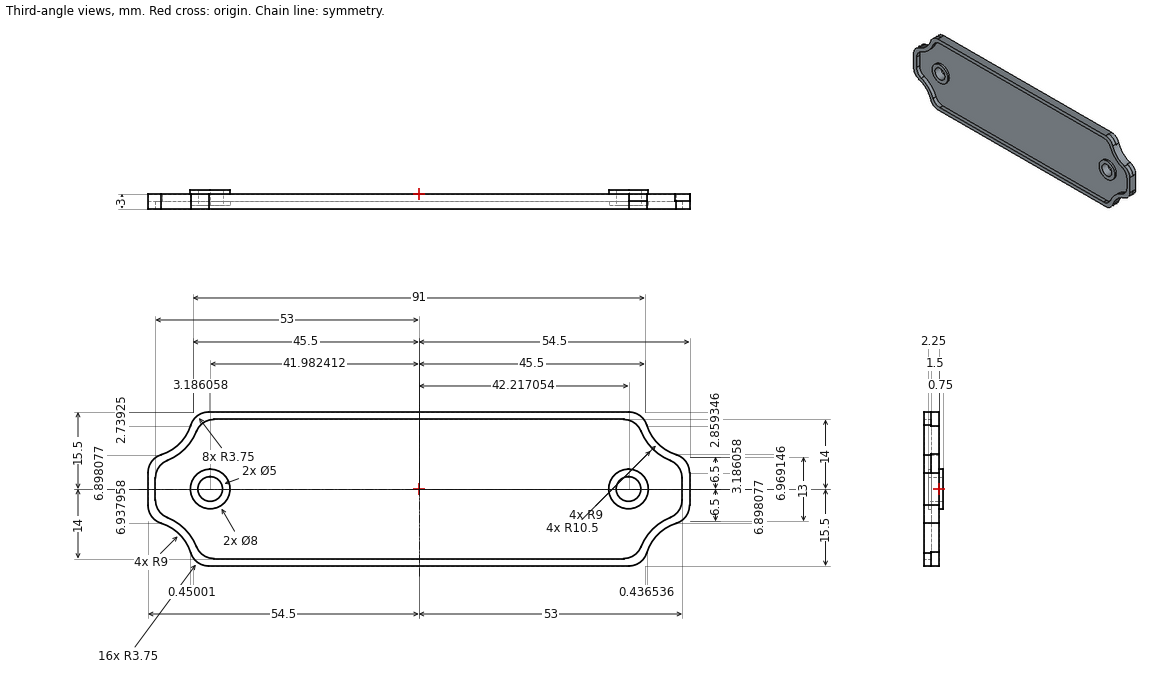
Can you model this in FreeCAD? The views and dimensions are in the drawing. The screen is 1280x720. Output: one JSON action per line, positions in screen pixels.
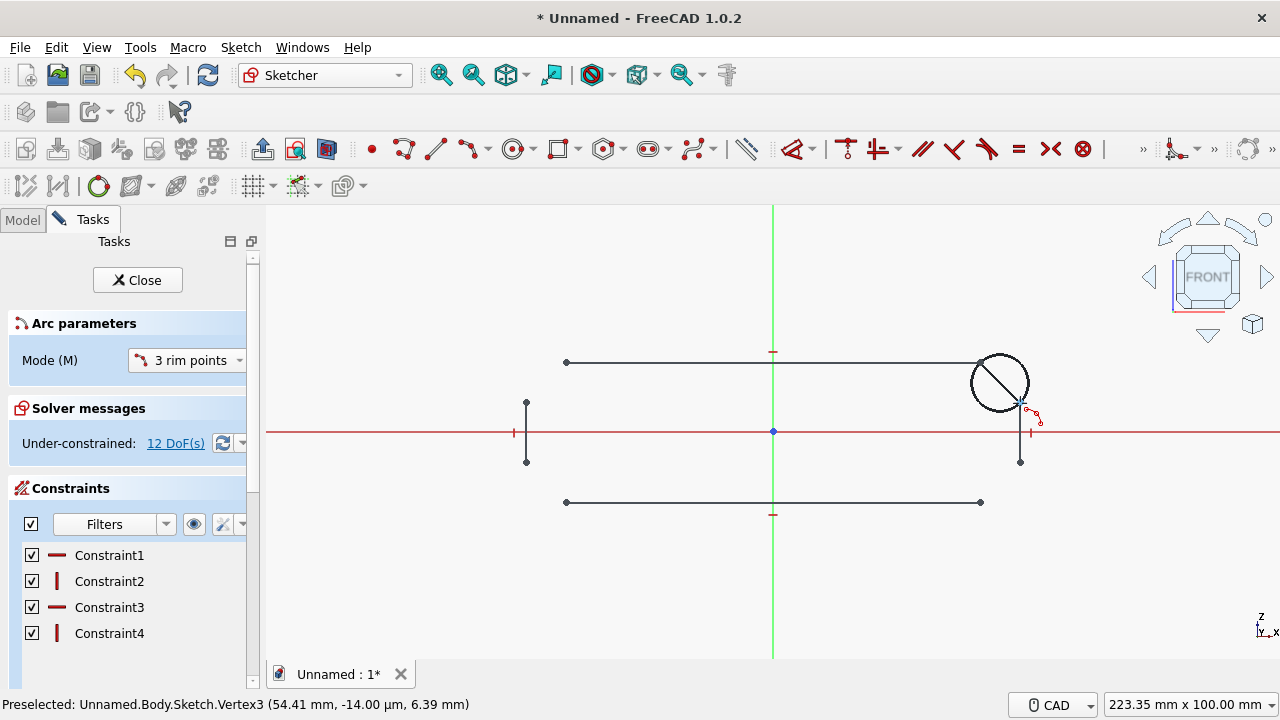
{"action": "scroll", "coordinate": [992, 391], "scroll_direction": "up", "scroll_amount": 2}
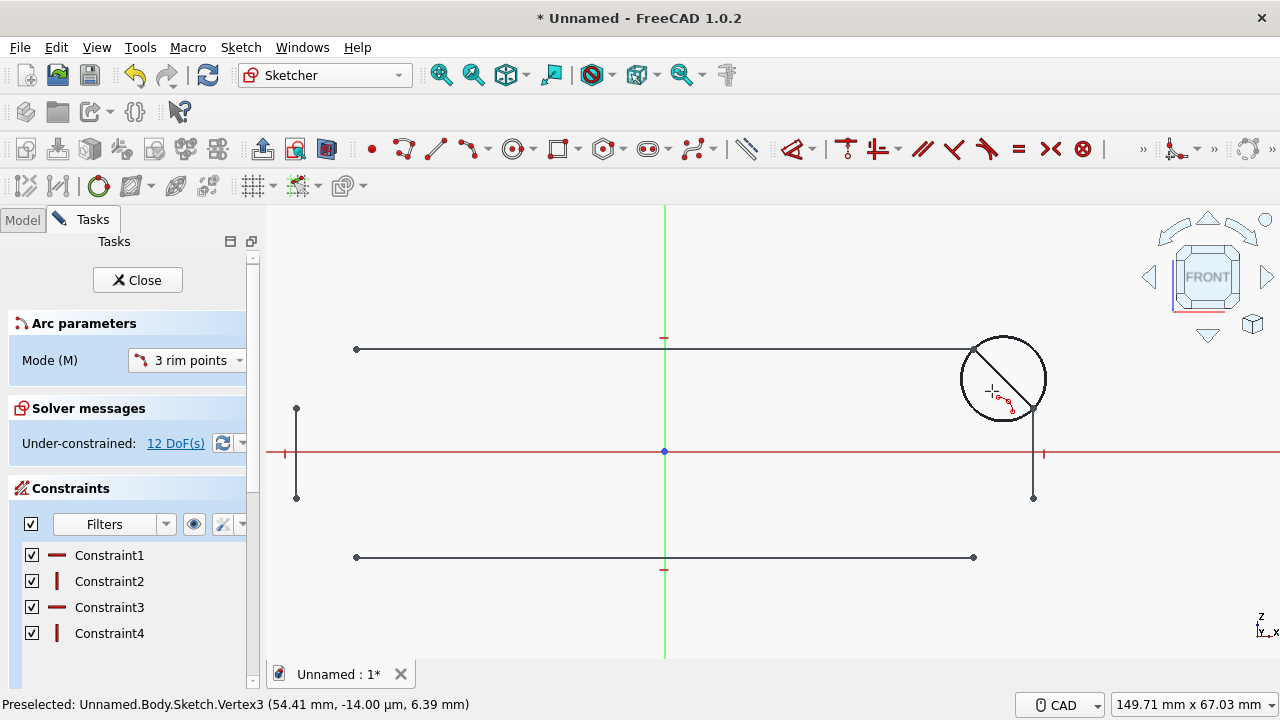
{"action": "left_click", "coordinate": [991, 390]}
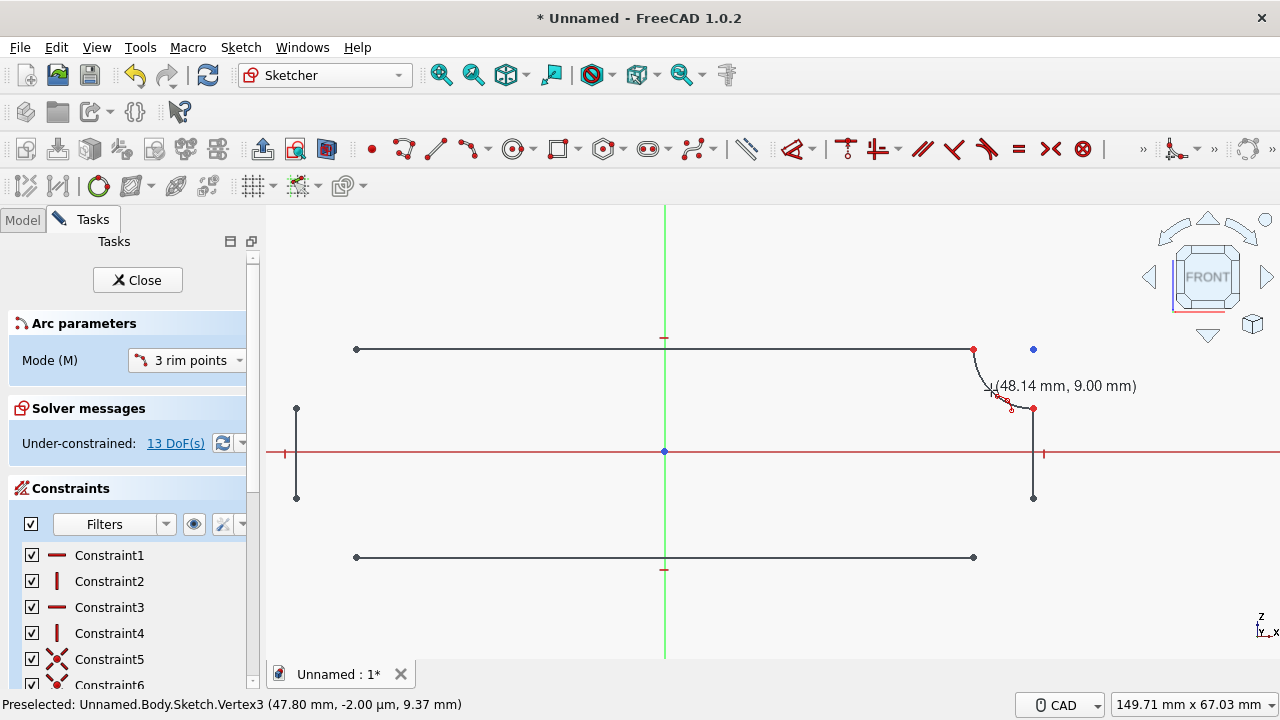
{"action": "left_click", "coordinate": [1033, 498]}
{"action": "left_click", "coordinate": [974, 558]}
{"action": "left_click", "coordinate": [991, 514]}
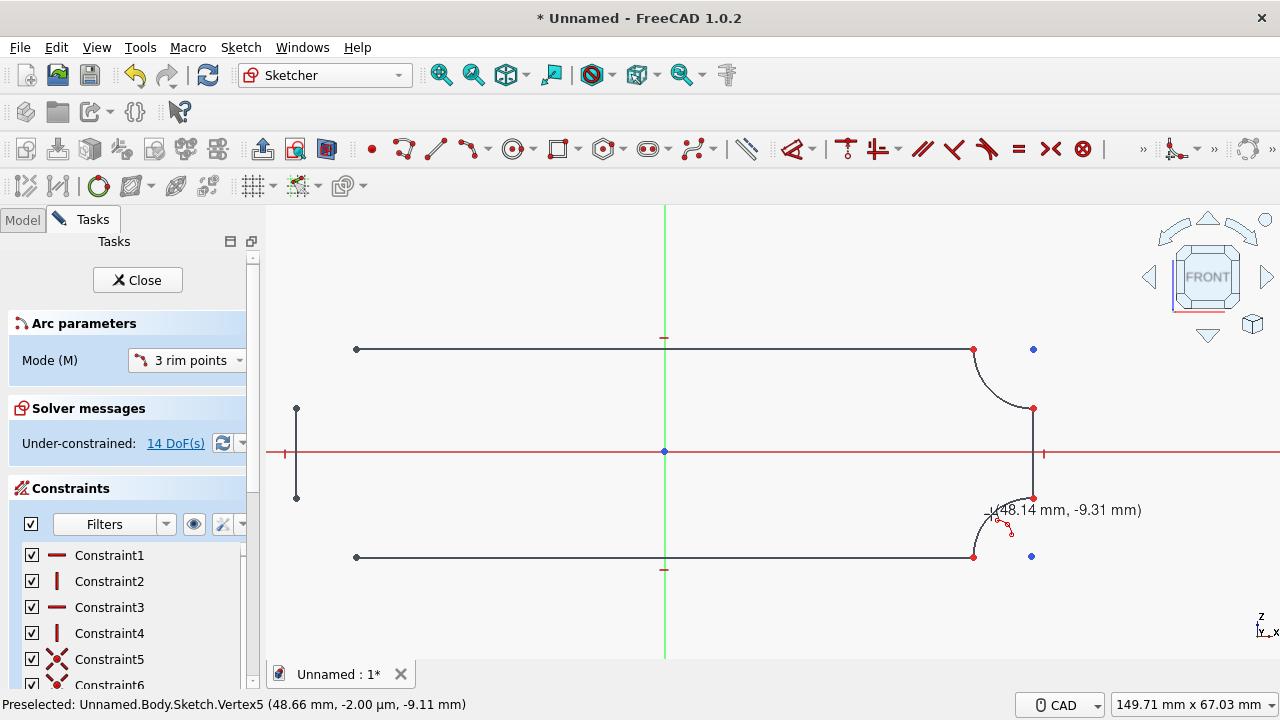
{"action": "left_click", "coordinate": [356, 558]}
{"action": "left_click", "coordinate": [296, 498]}
{"action": "left_click", "coordinate": [339, 514]}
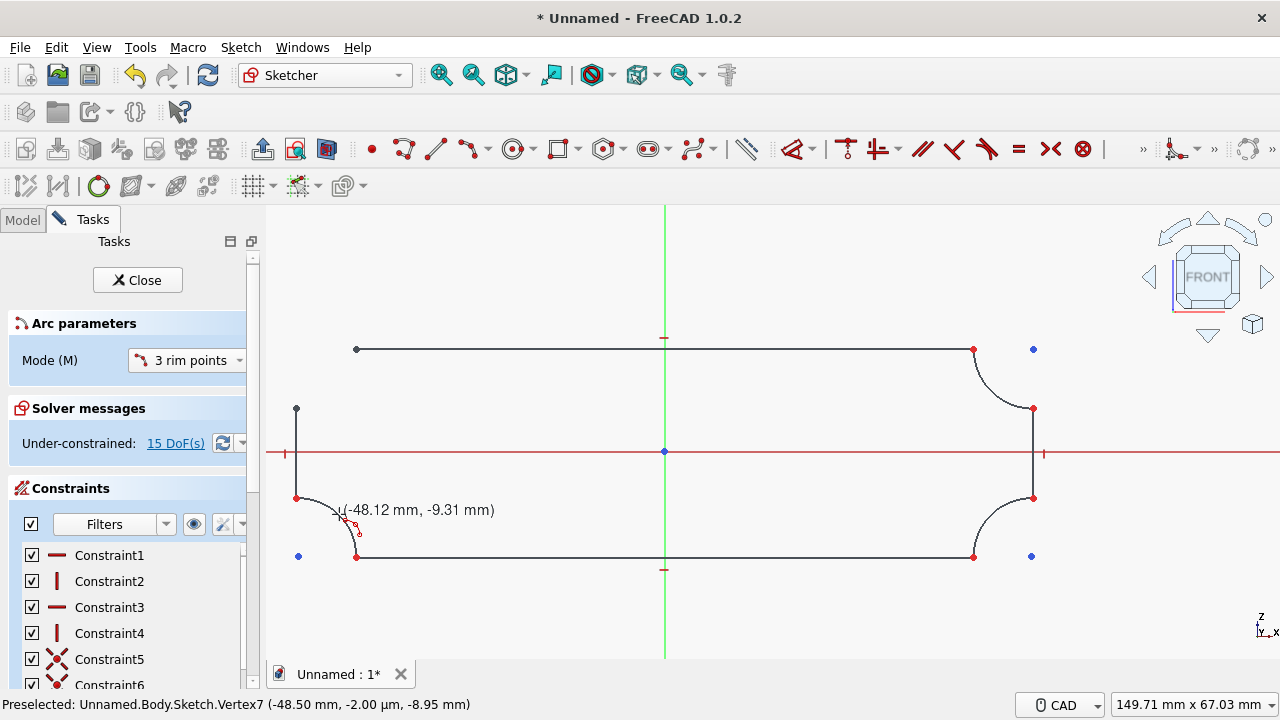
{"action": "left_click", "coordinate": [296, 409]}
{"action": "left_click", "coordinate": [356, 349]}
{"action": "left_click", "coordinate": [339, 390]}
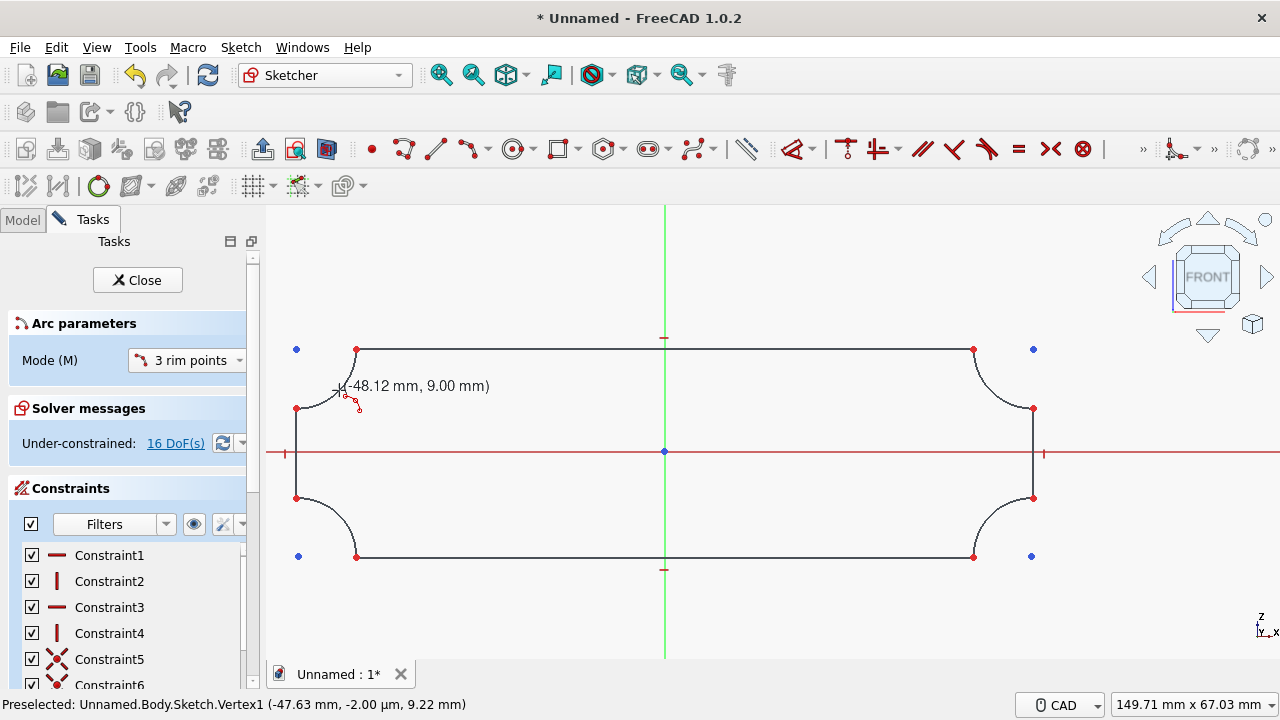
{"action": "left_click", "coordinate": [514, 150]}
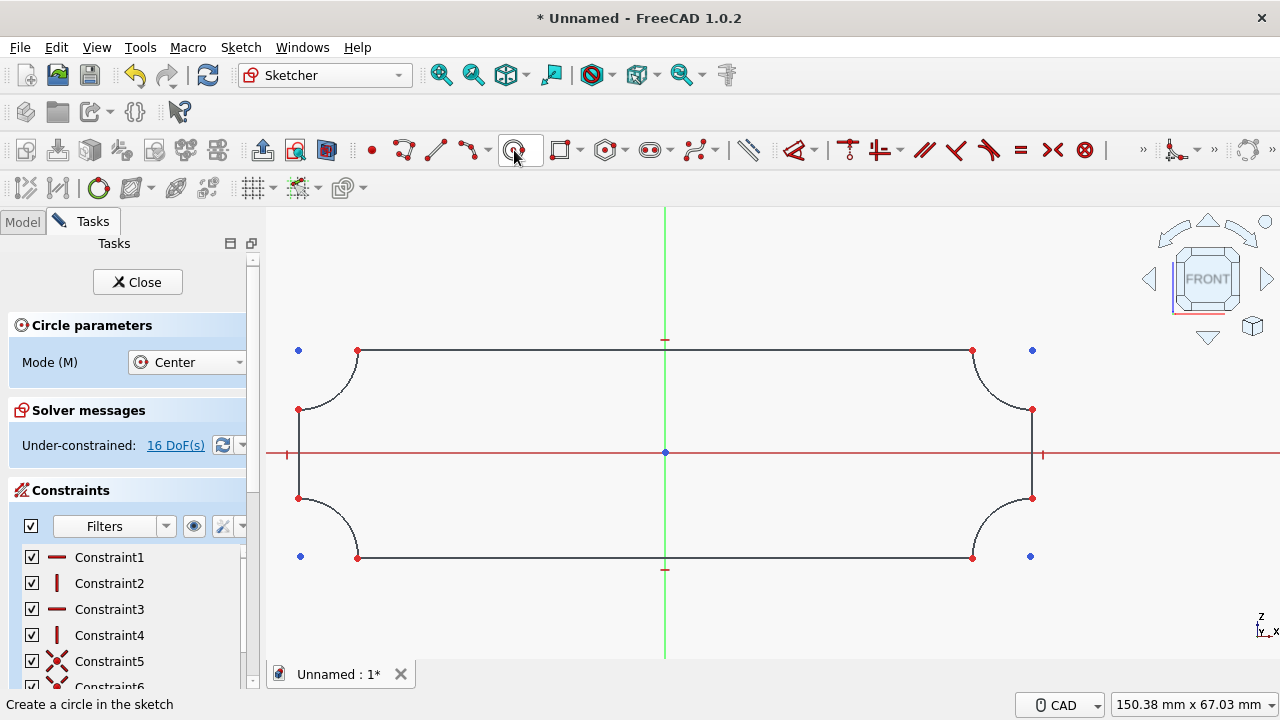
{"action": "scroll", "coordinate": [382, 453], "scroll_direction": "up", "scroll_amount": 2}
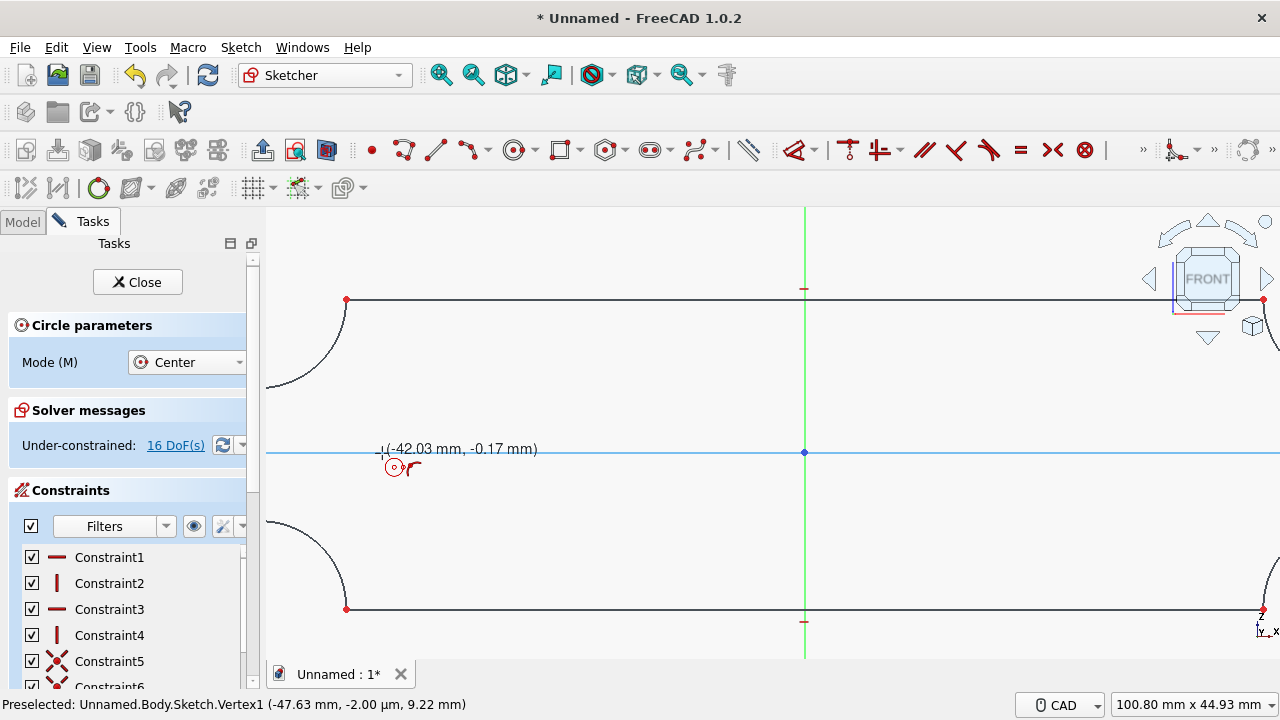
{"action": "left_click", "coordinate": [382, 453]}
{"action": "mouse_move", "coordinate": [400, 435]}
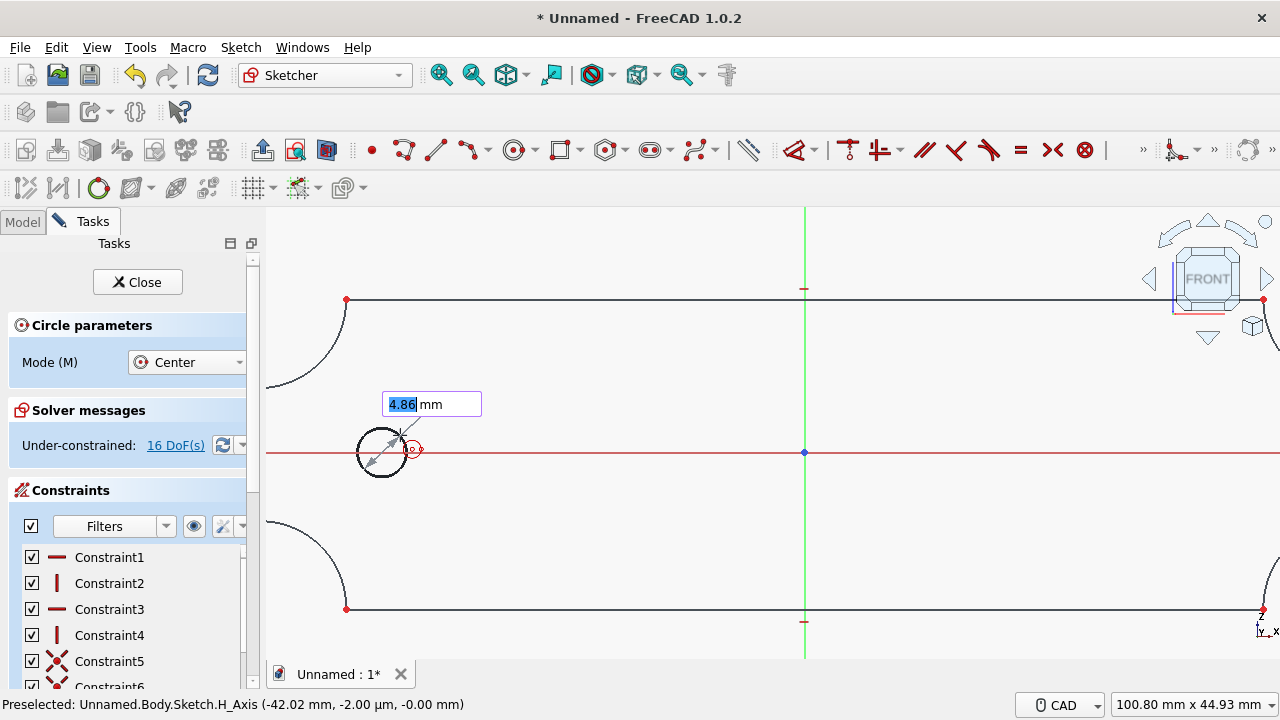
{"action": "type", "text": "5"}
{"action": "key", "text": "Return"}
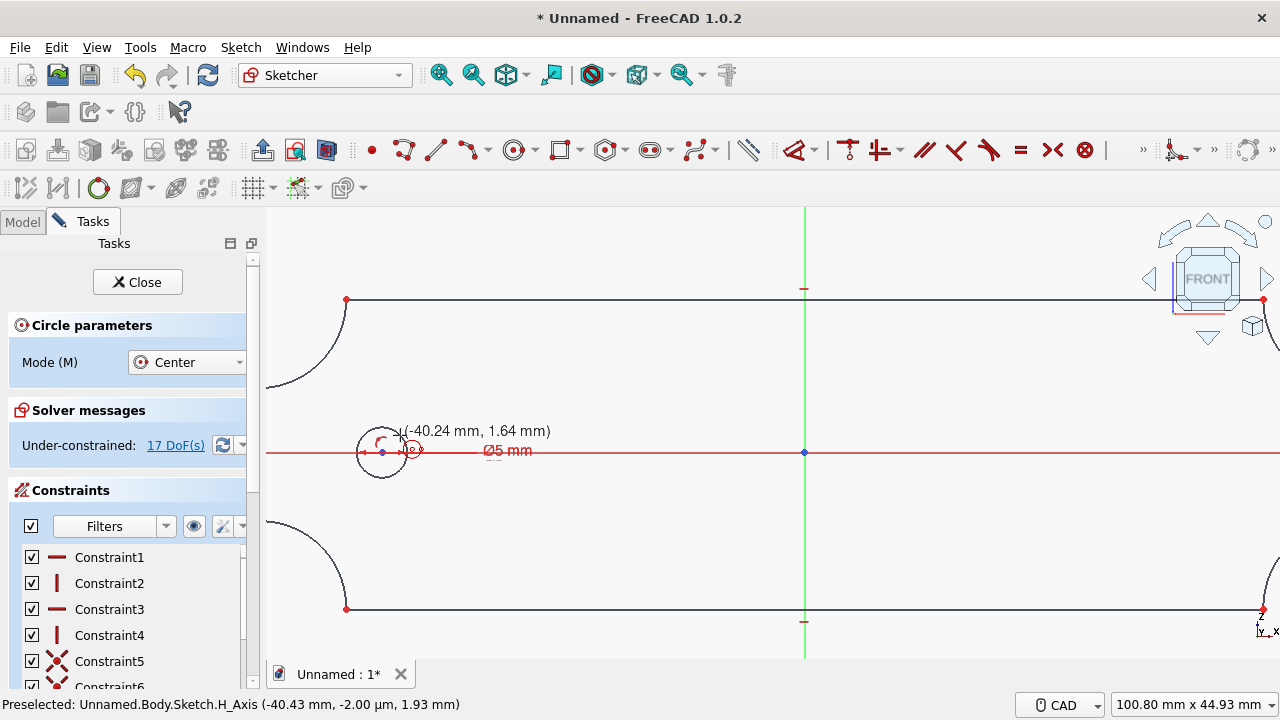
{"action": "scroll", "coordinate": [583, 409], "scroll_direction": "down", "scroll_amount": 3}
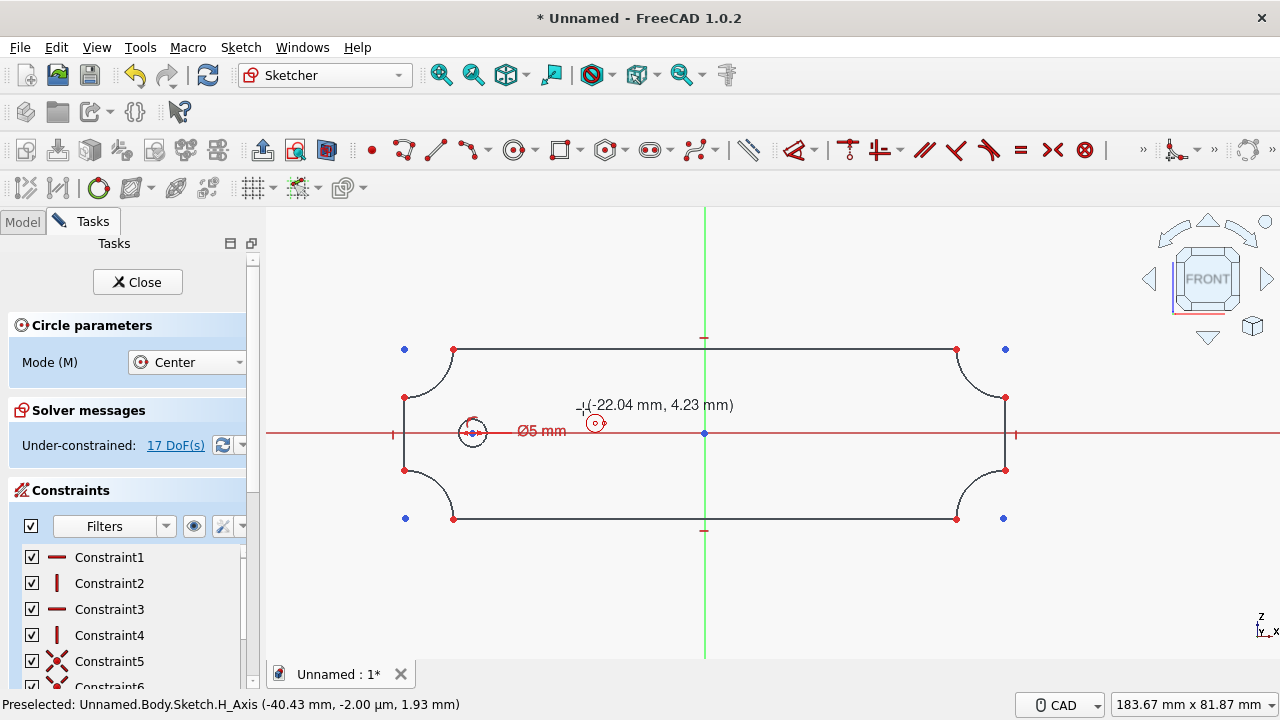
{"action": "scroll", "coordinate": [938, 433], "scroll_direction": "up", "scroll_amount": 3}